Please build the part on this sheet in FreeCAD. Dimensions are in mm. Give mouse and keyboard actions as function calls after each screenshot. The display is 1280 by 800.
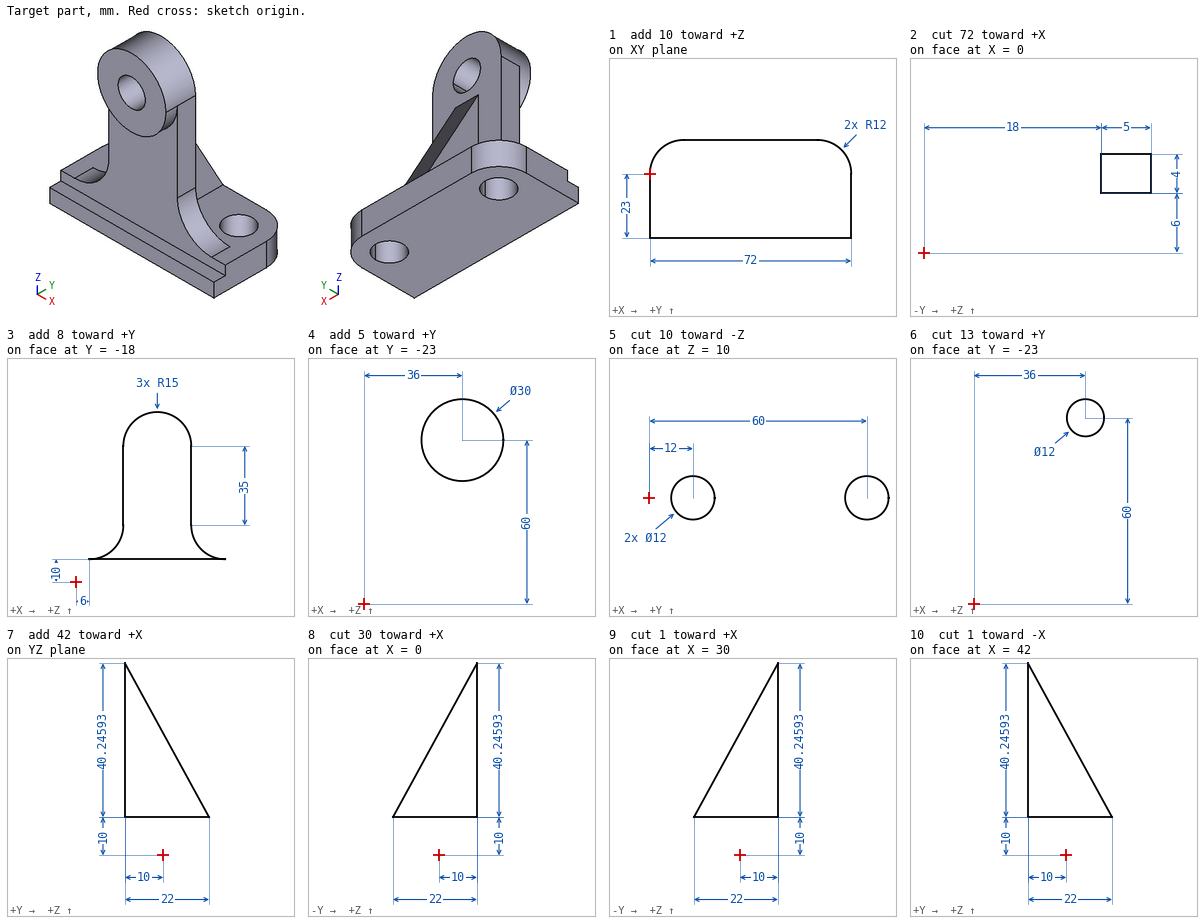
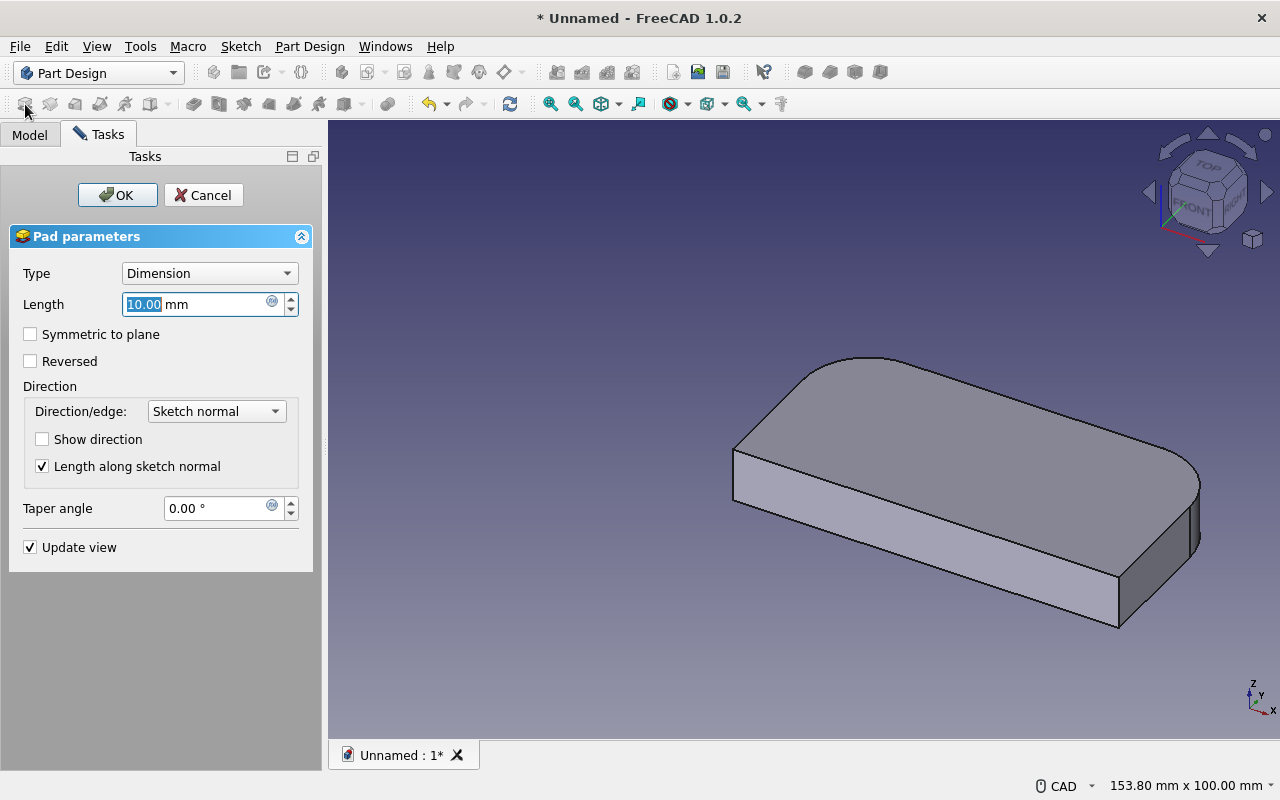
text(10)
key(Tab)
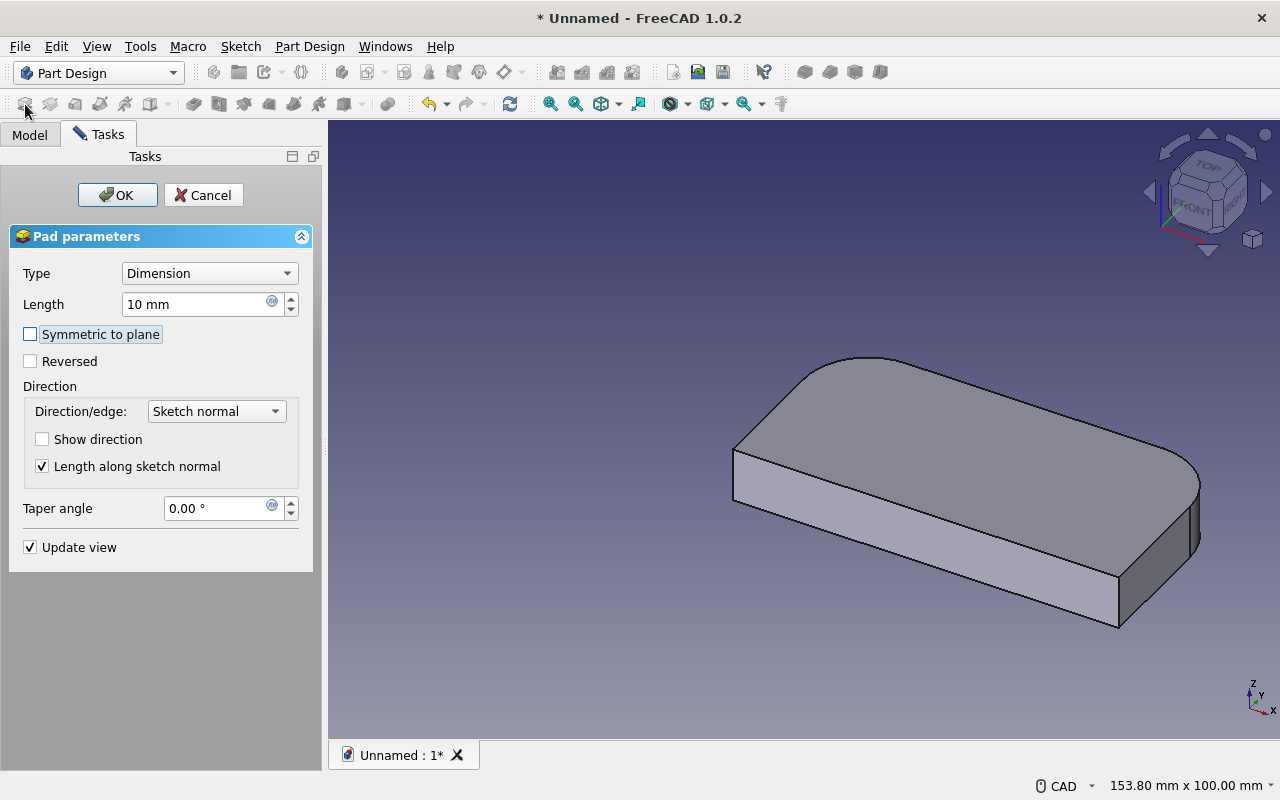
click(118, 195)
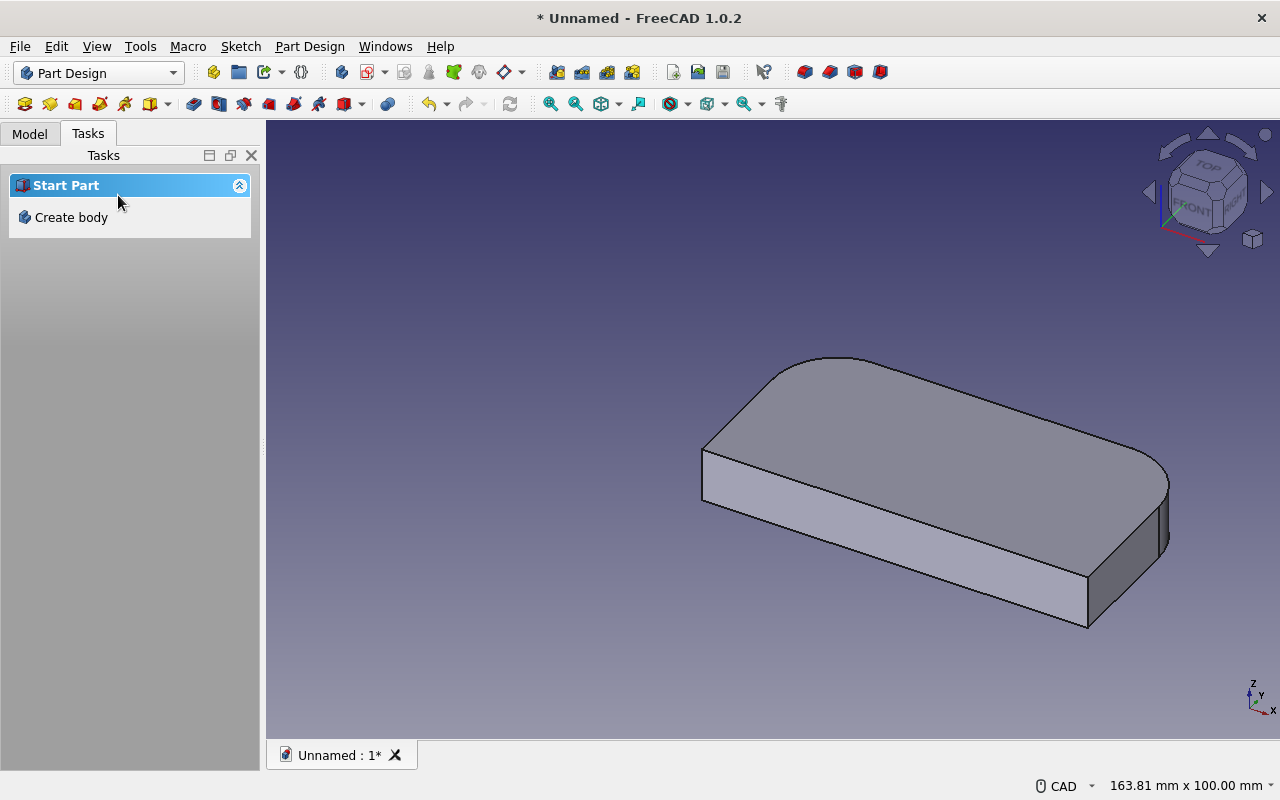
key(6)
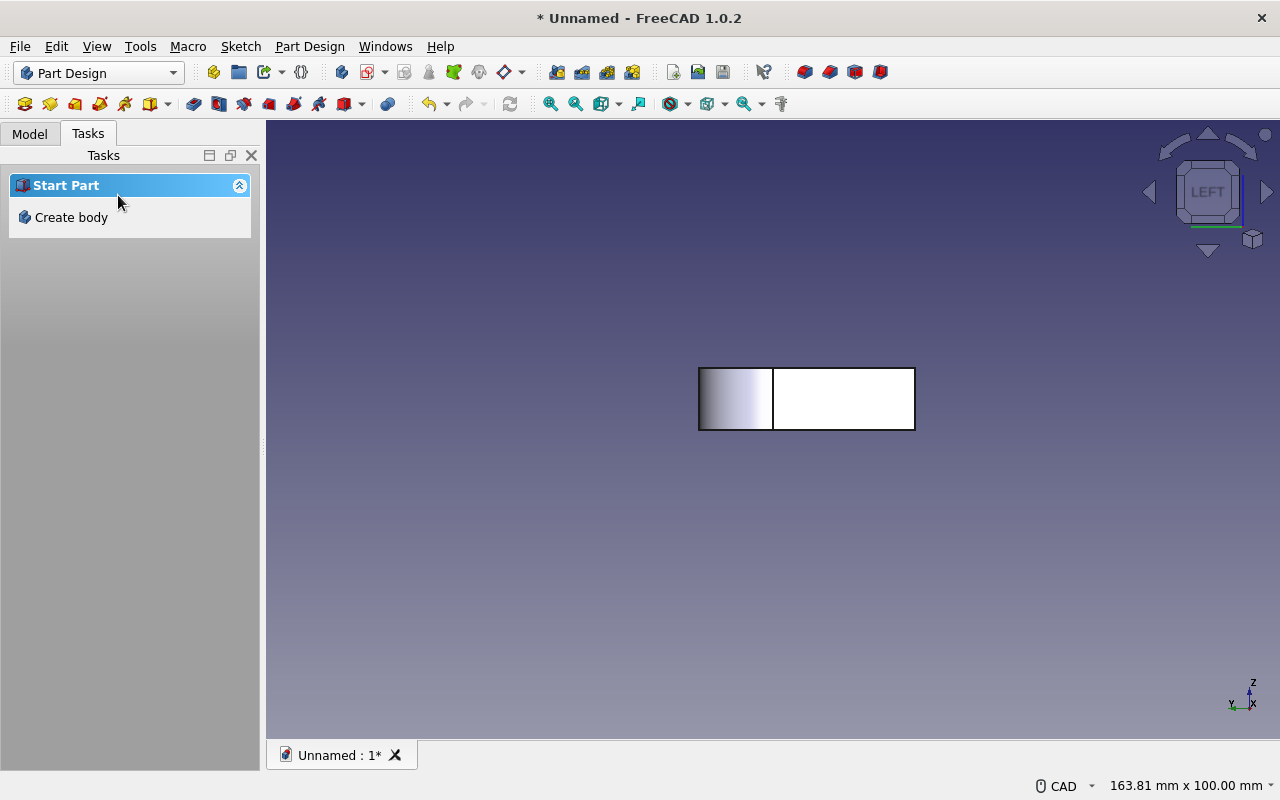
key(v)
key(f)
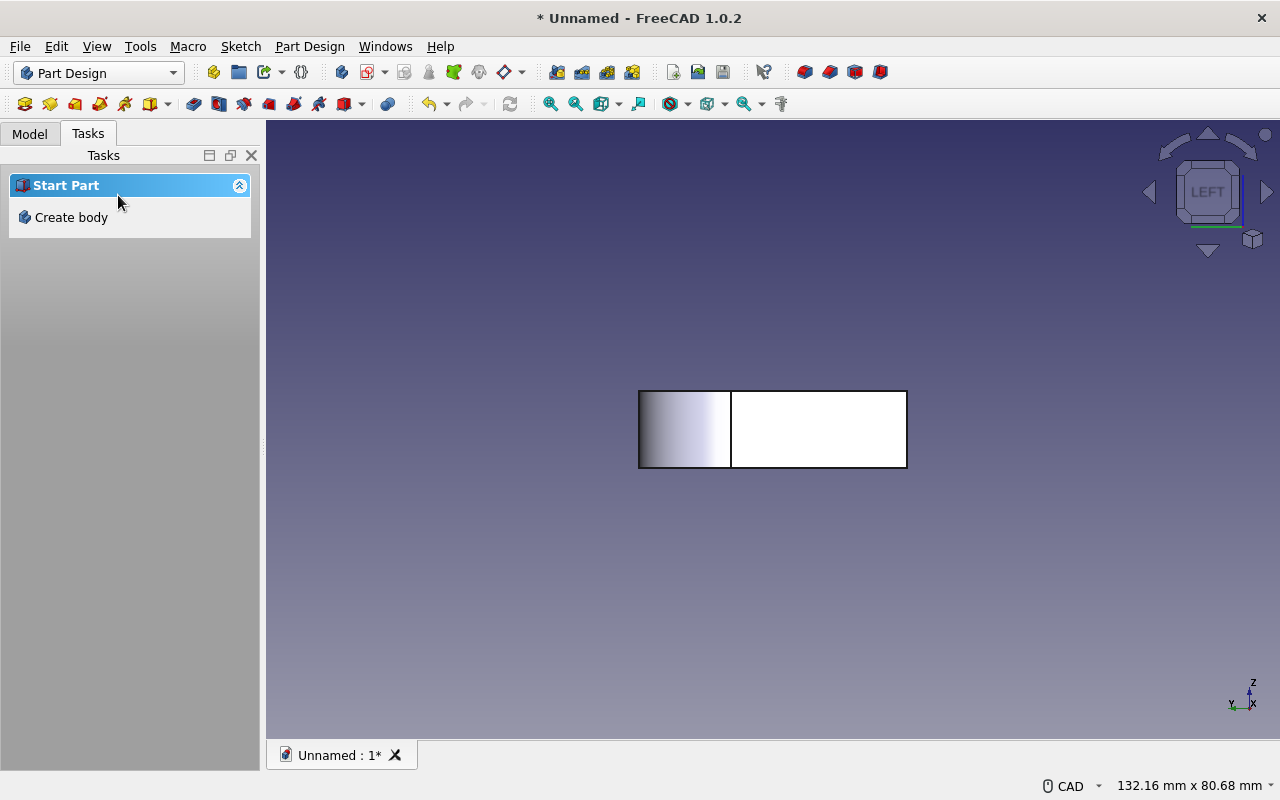
click(794, 428)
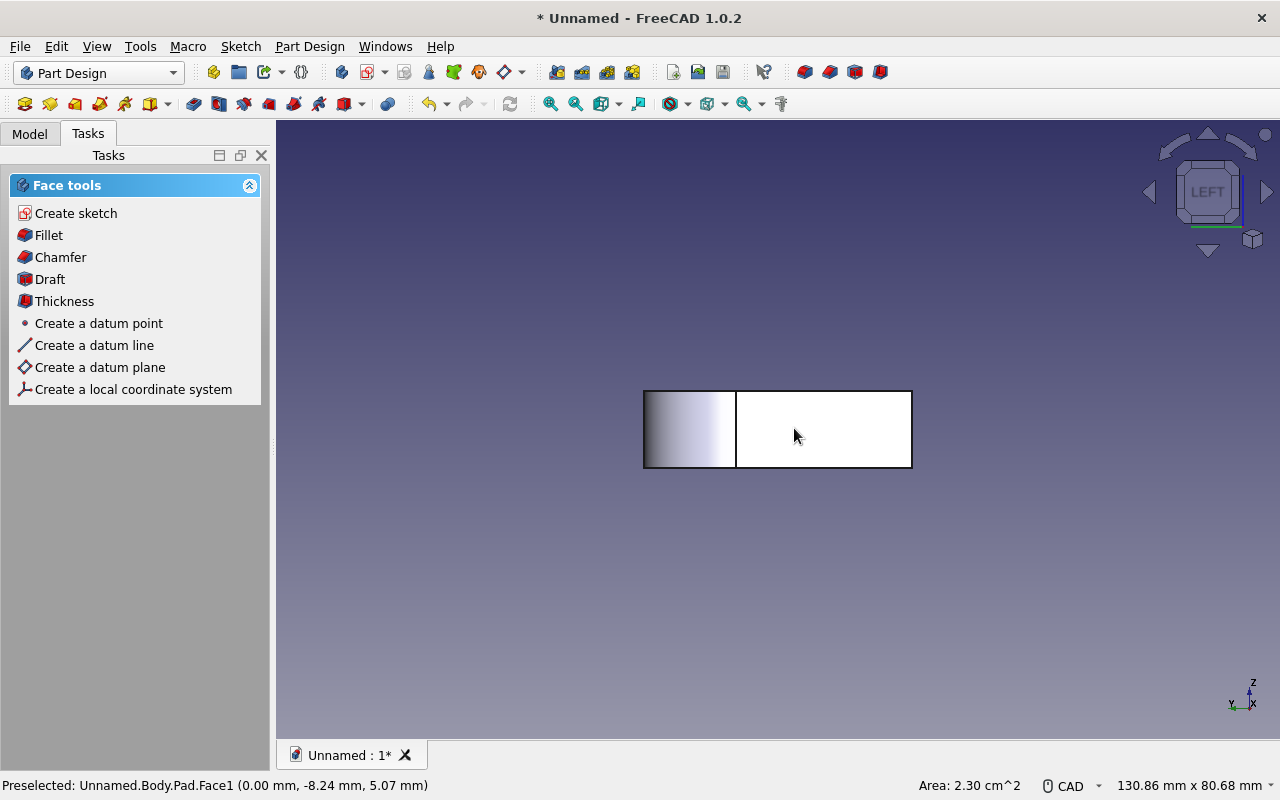
click(366, 72)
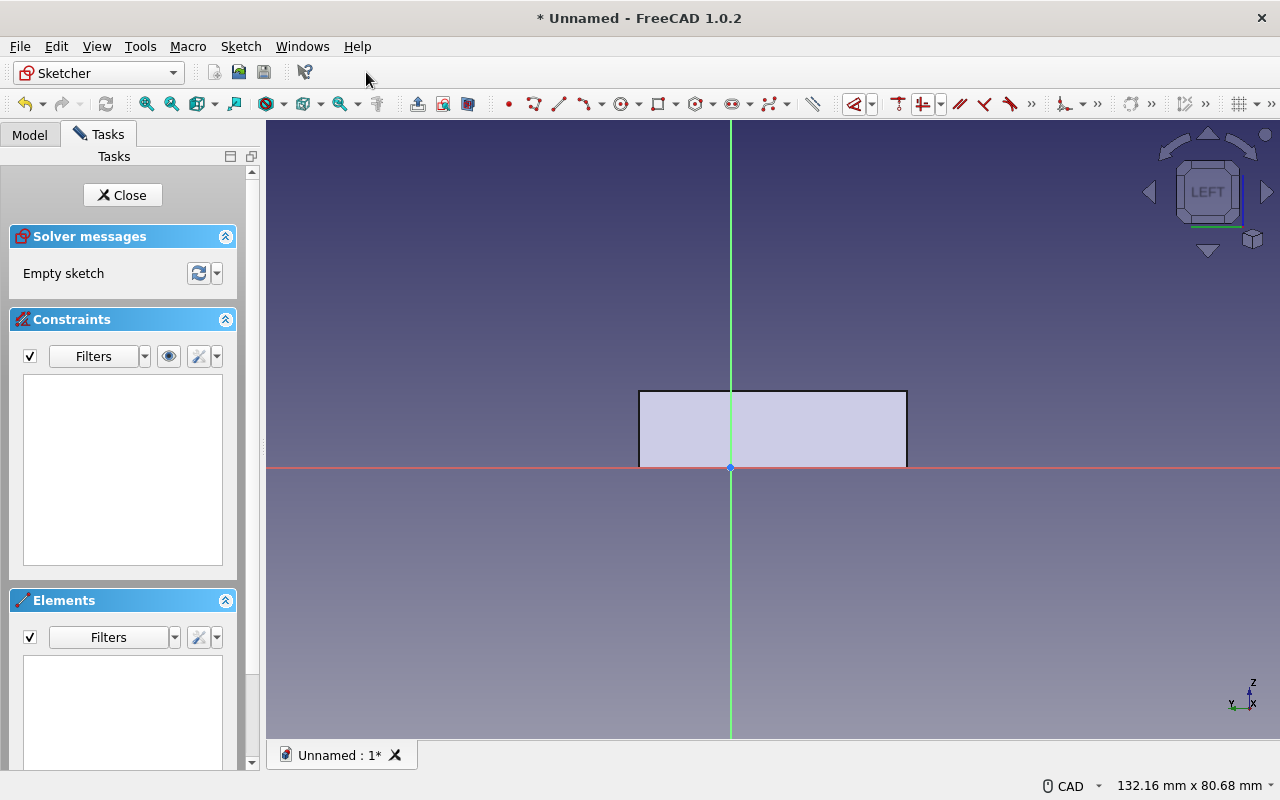
scroll(903, 405, up, 13)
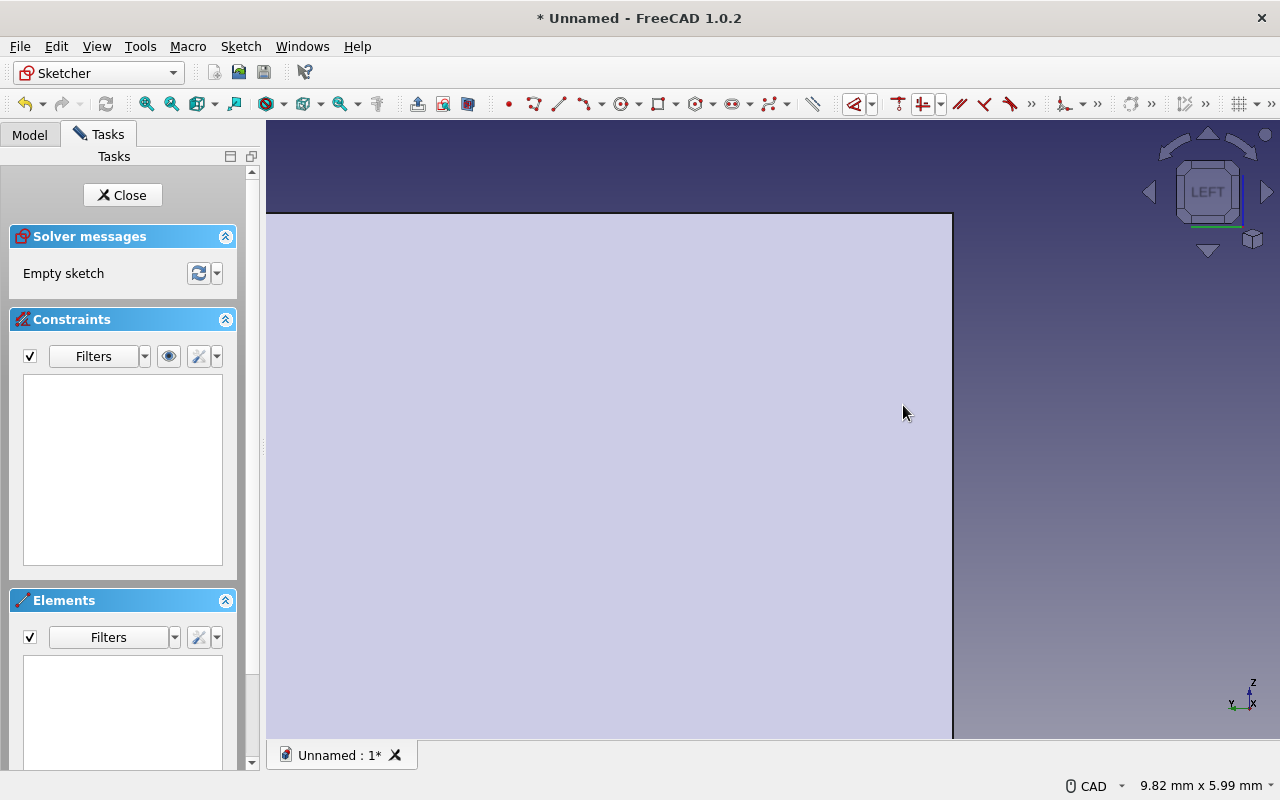
click(658, 104)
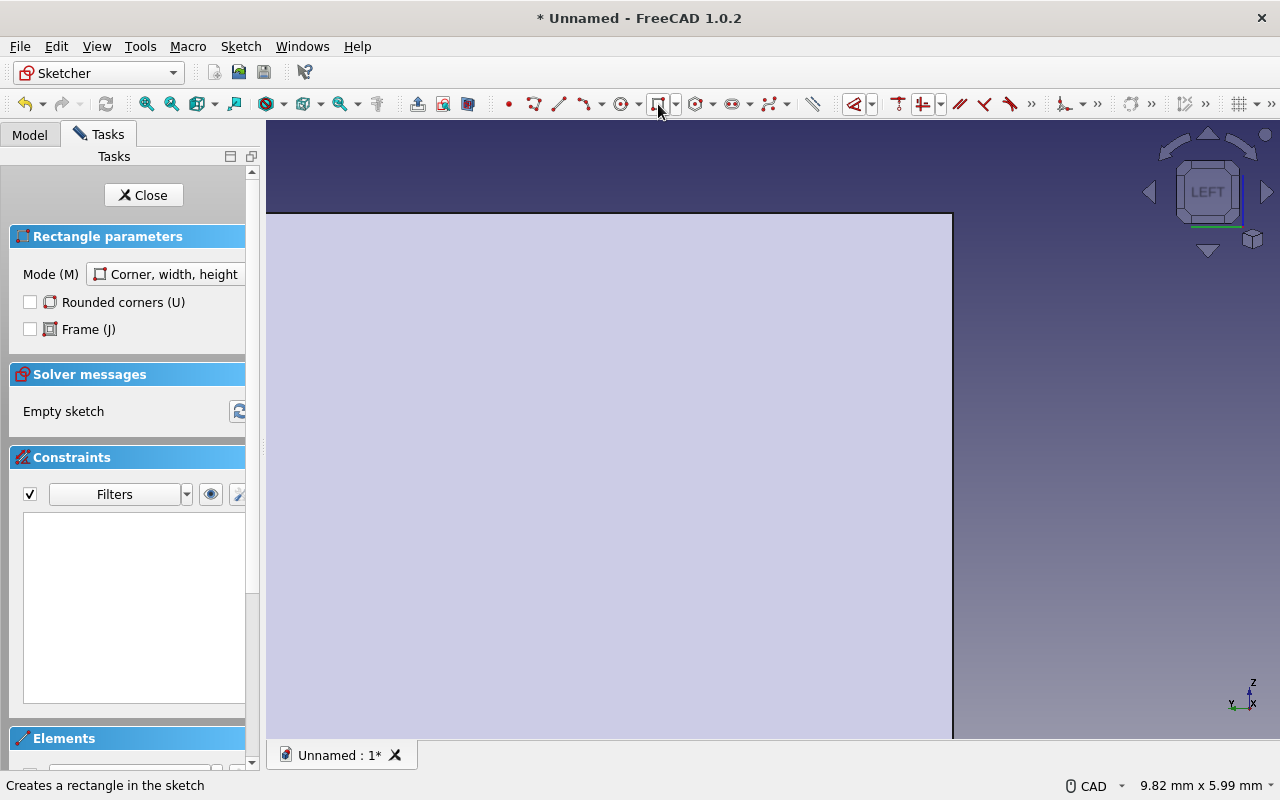
click(436, 213)
move(953, 626)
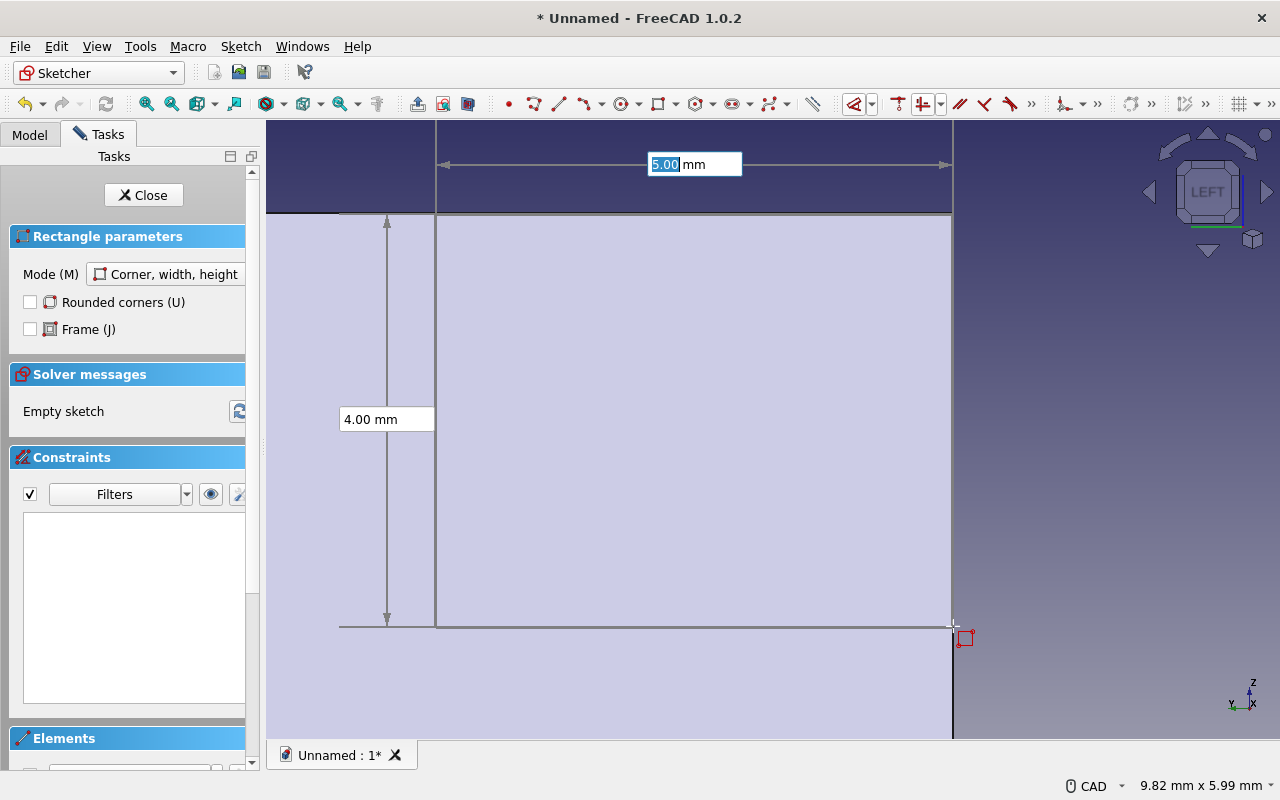
text(5)
key(Tab)
text(4)
key(Return)
key(Escape)